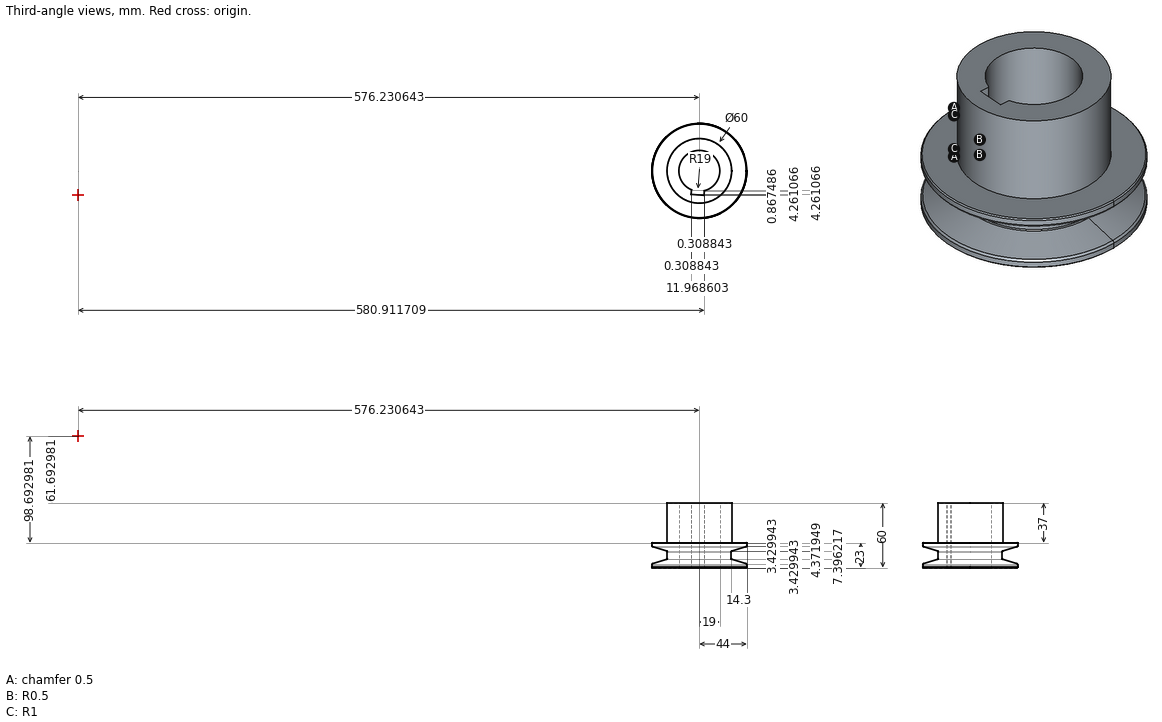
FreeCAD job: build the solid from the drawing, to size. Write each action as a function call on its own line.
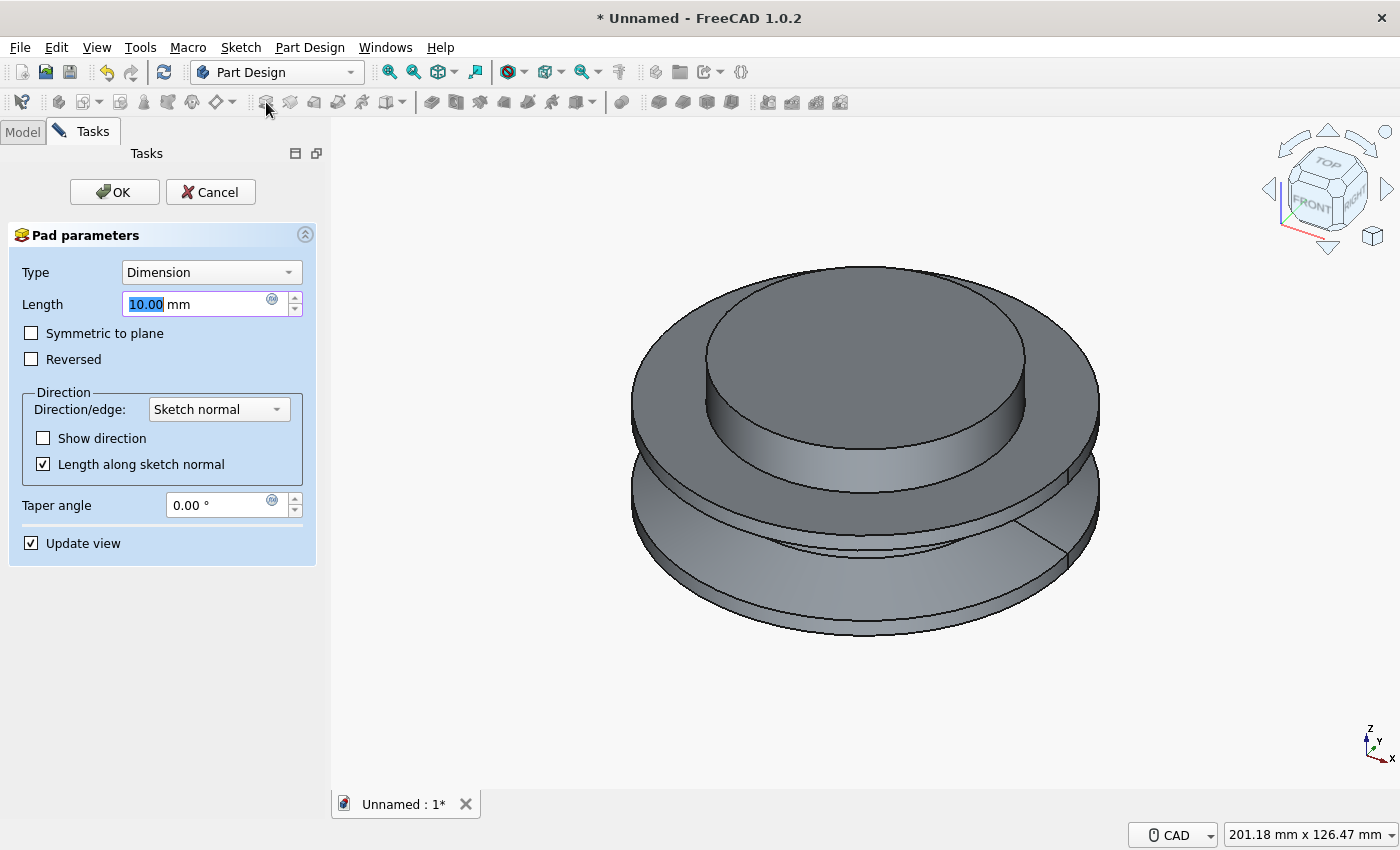
text(37)
key(Tab)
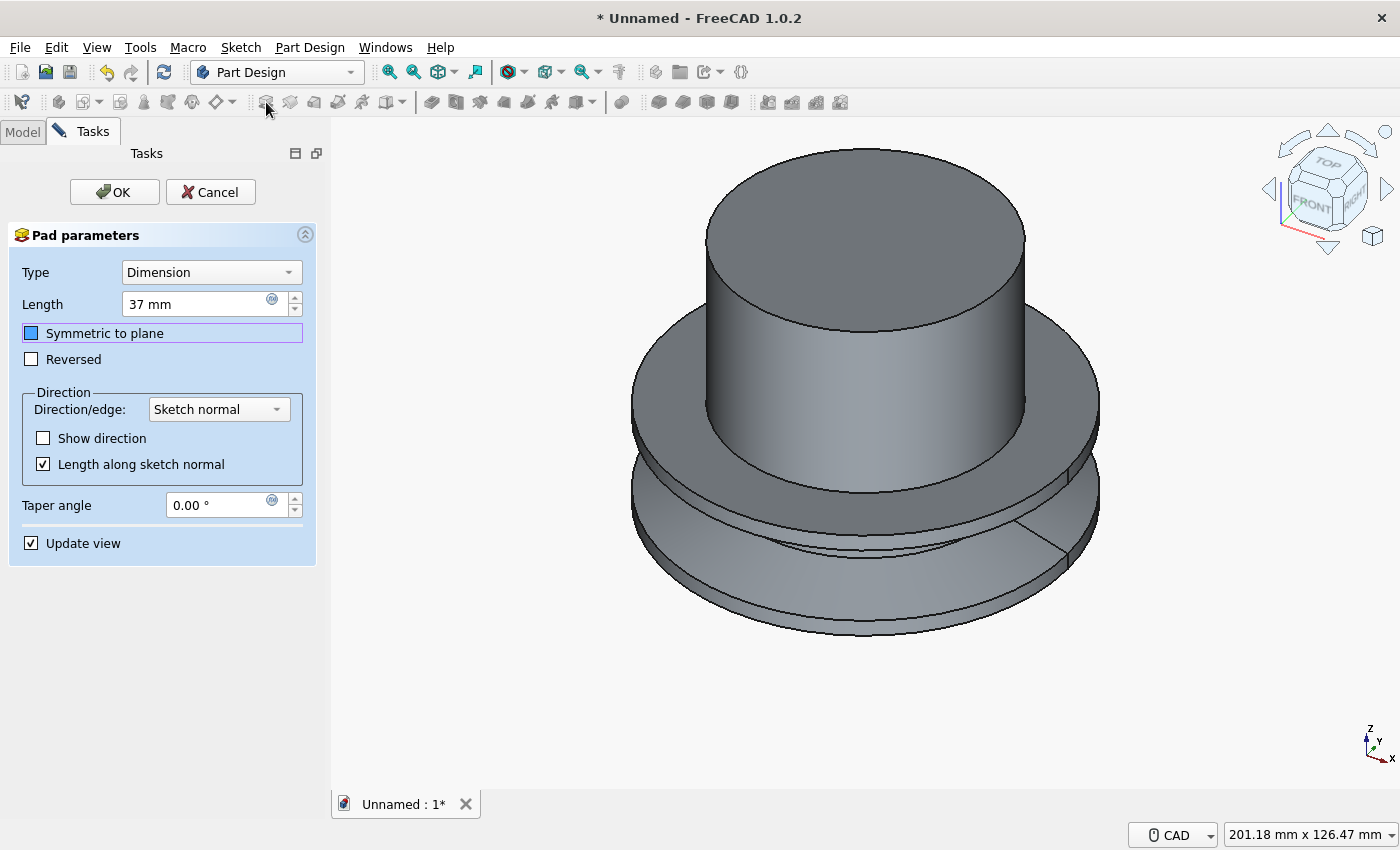
click(115, 192)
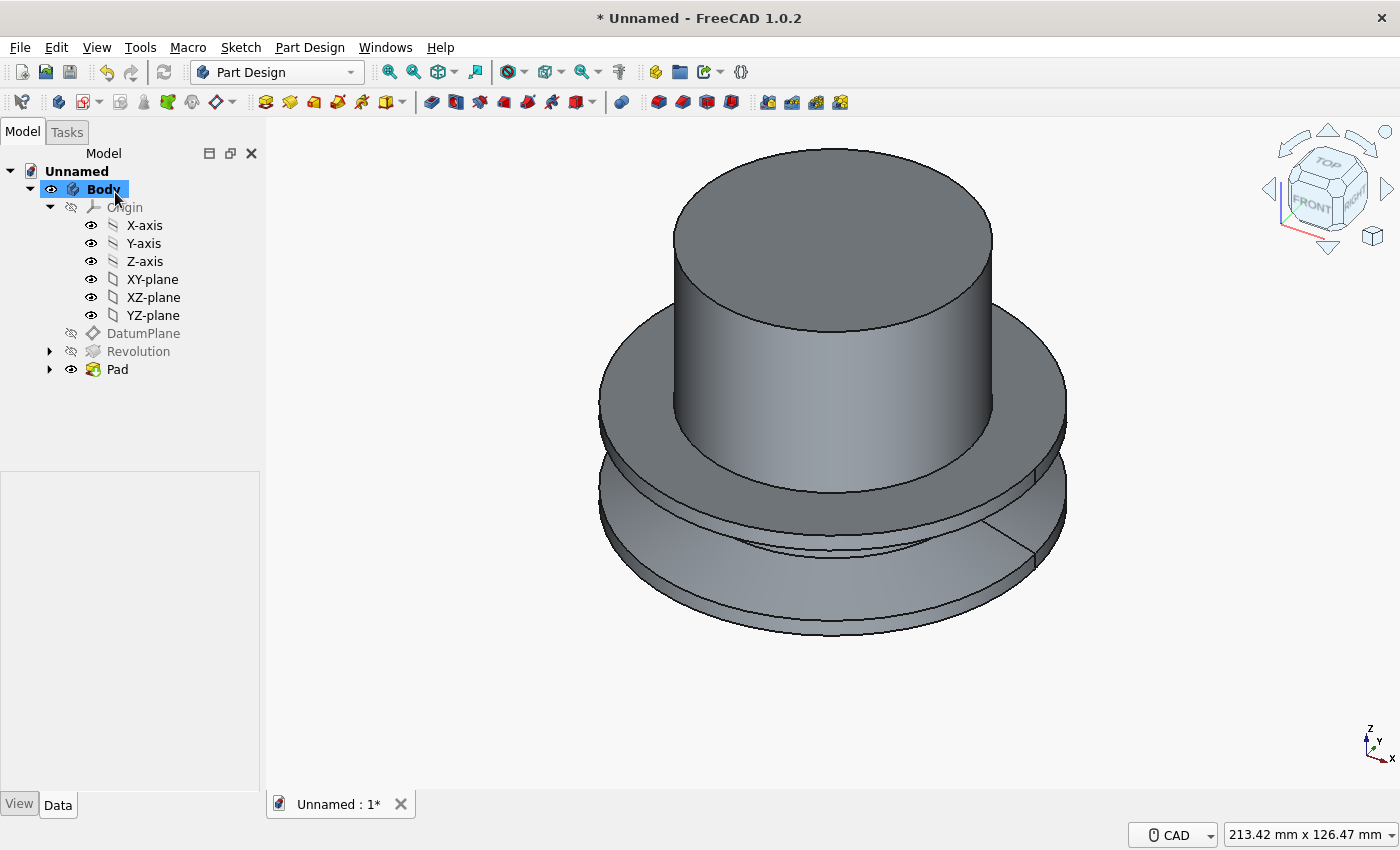
click(390, 72)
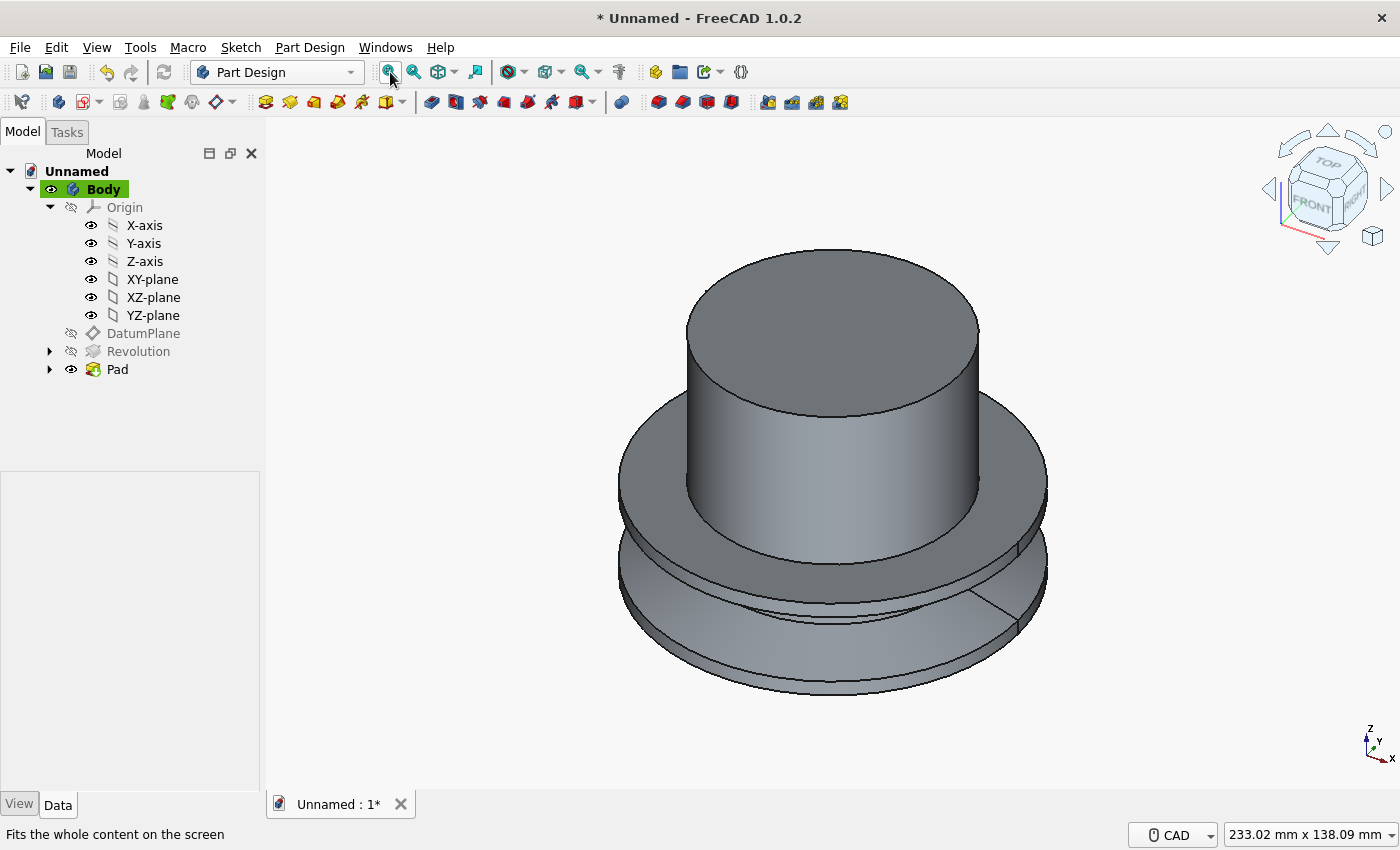
key(5)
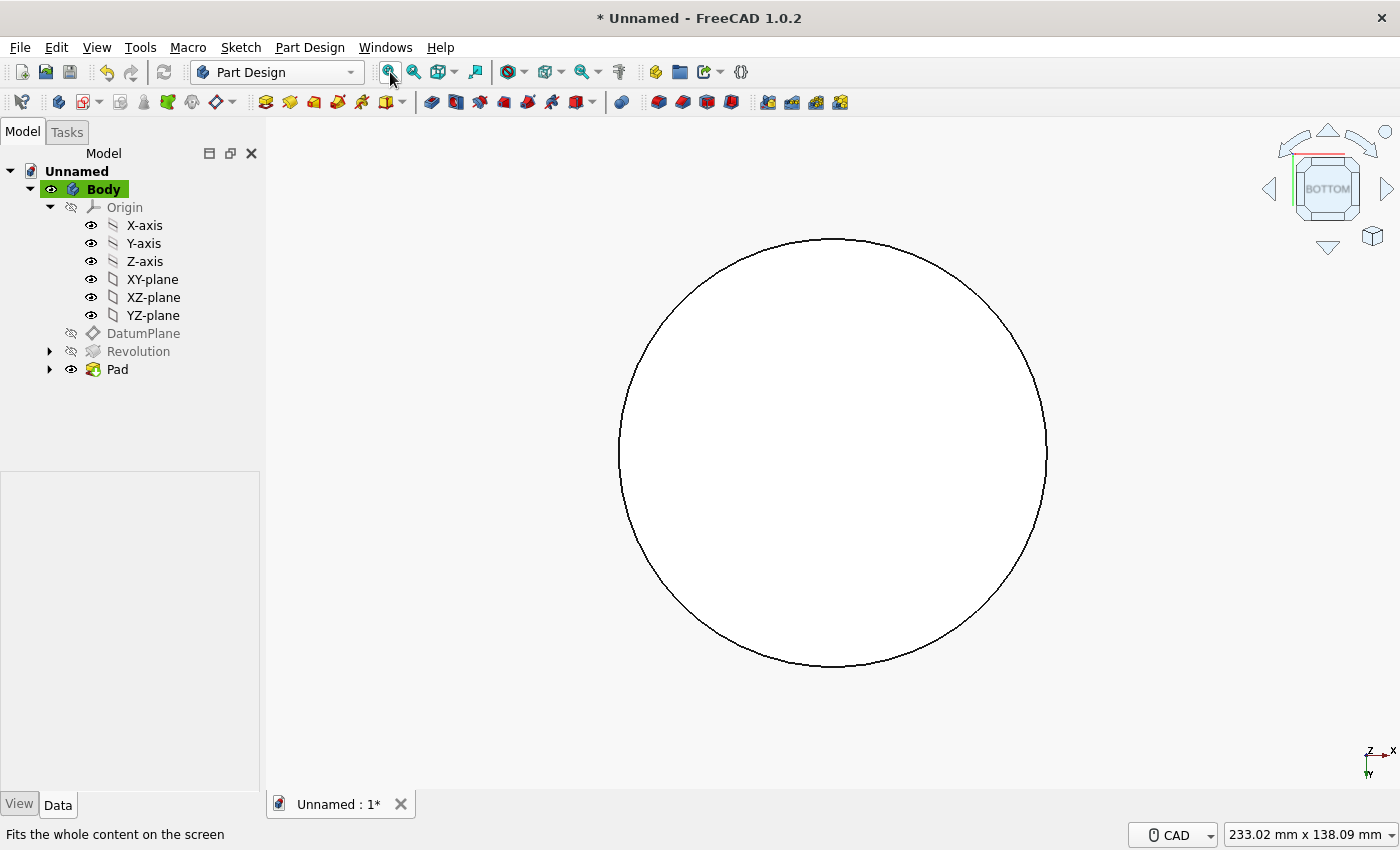
click(833, 452)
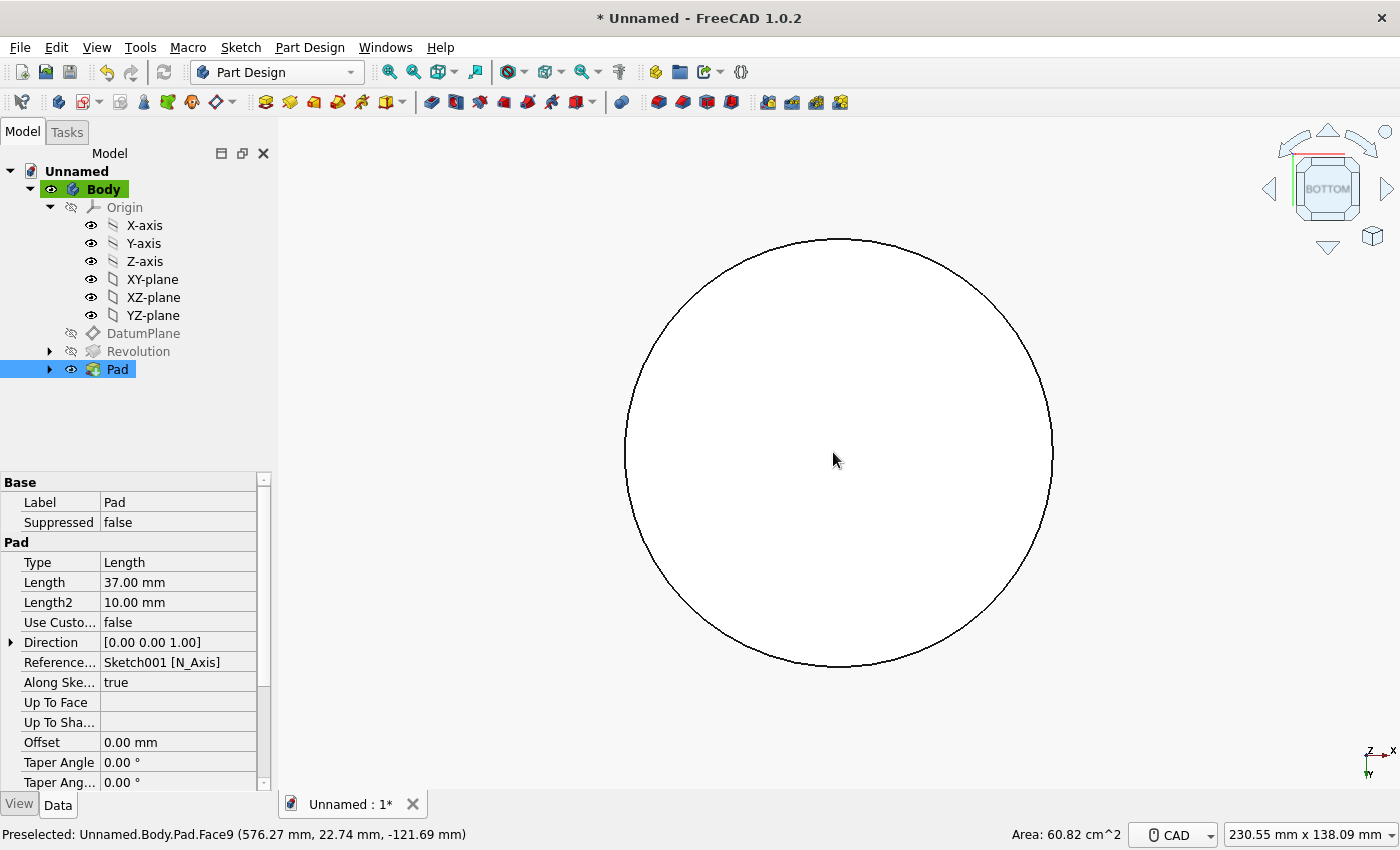
click(84, 102)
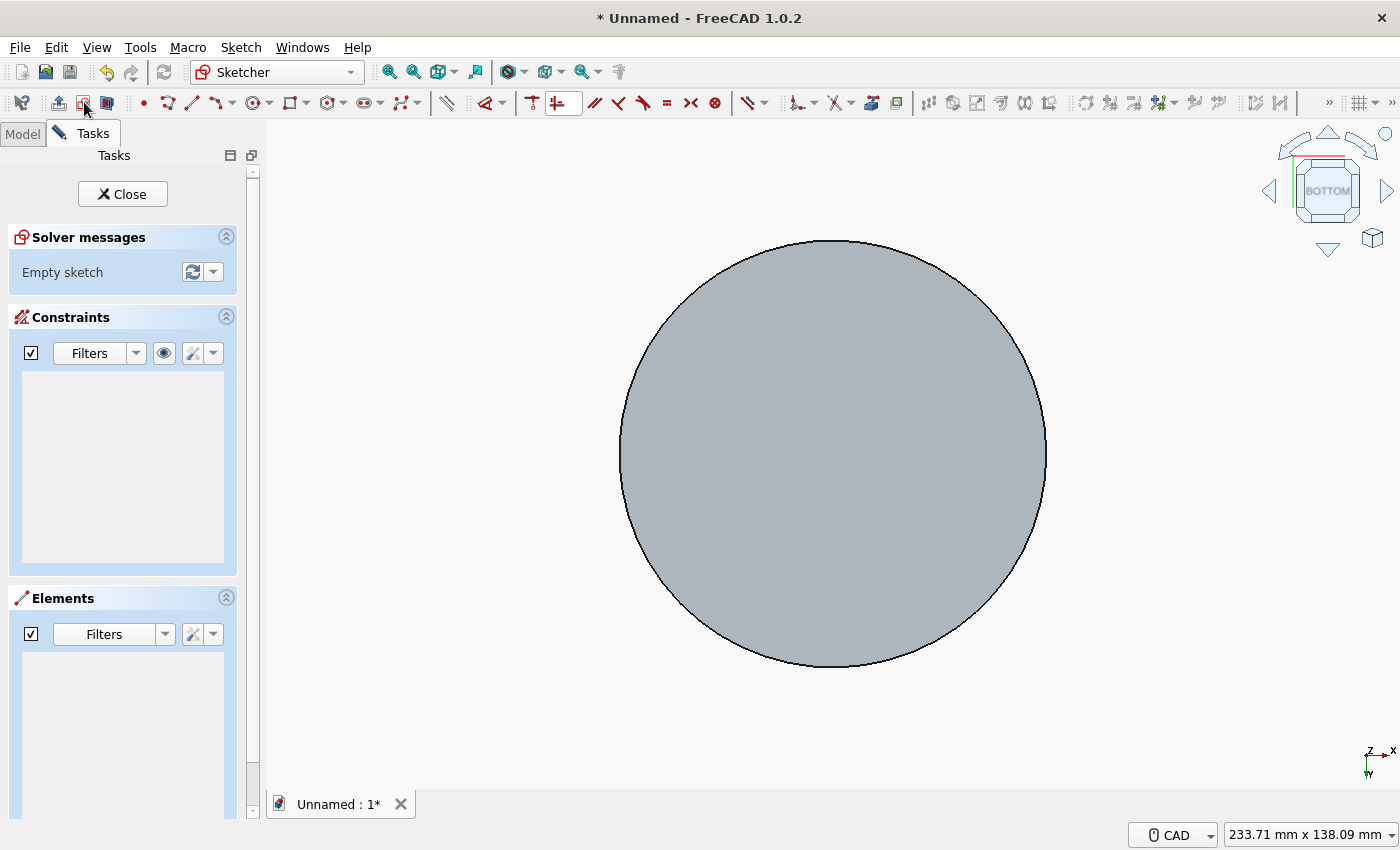
scroll(832, 347, up, 12)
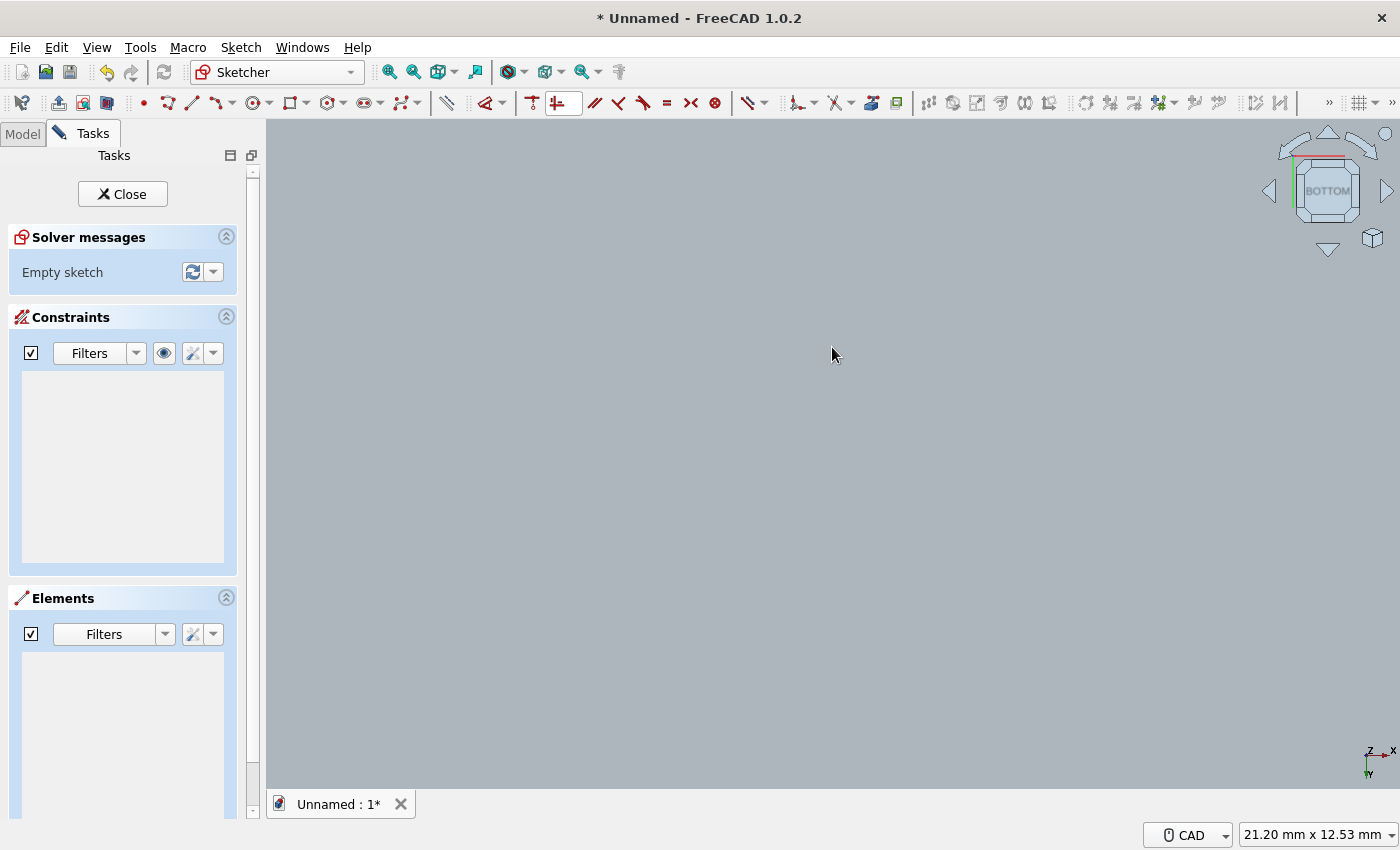
click(168, 104)